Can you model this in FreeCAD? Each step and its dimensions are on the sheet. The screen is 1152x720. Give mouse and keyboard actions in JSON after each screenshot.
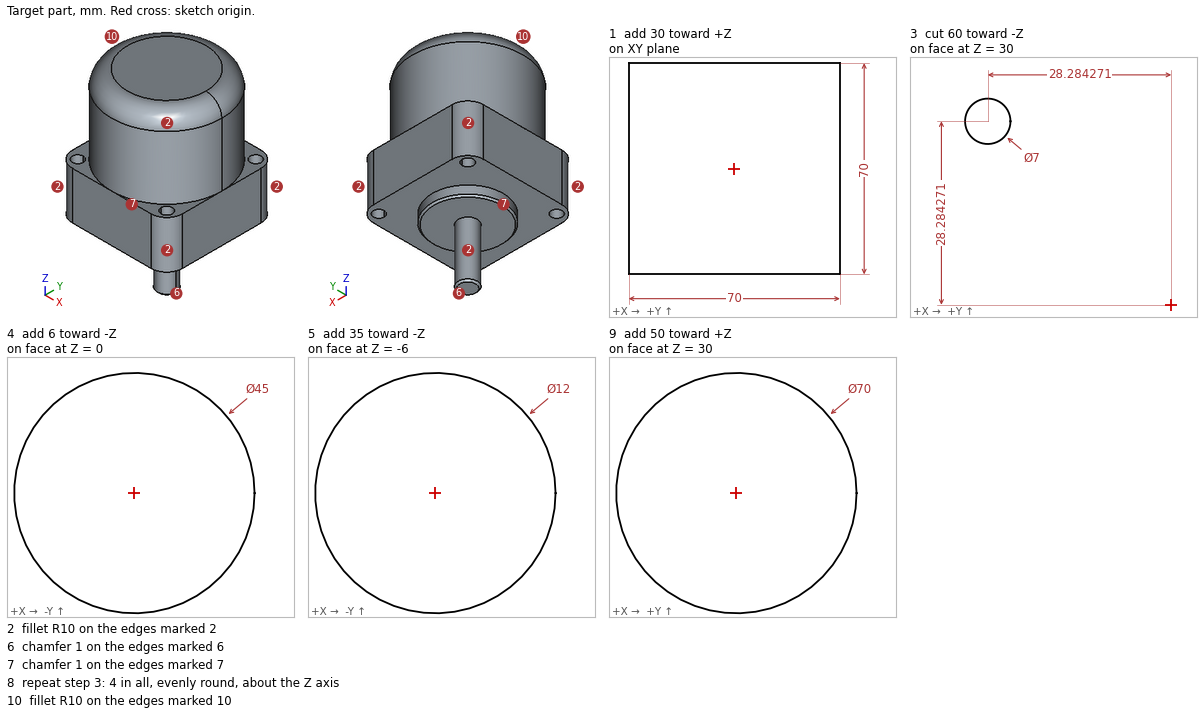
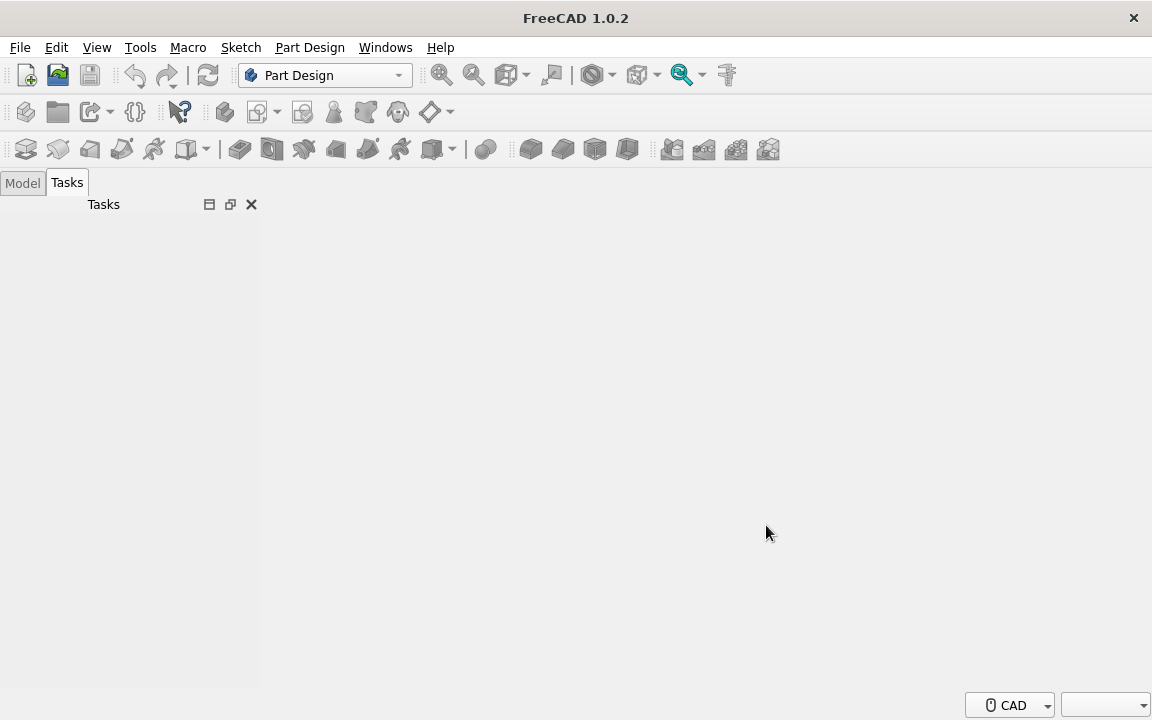
{"action": "key", "text": "ctrl+n"}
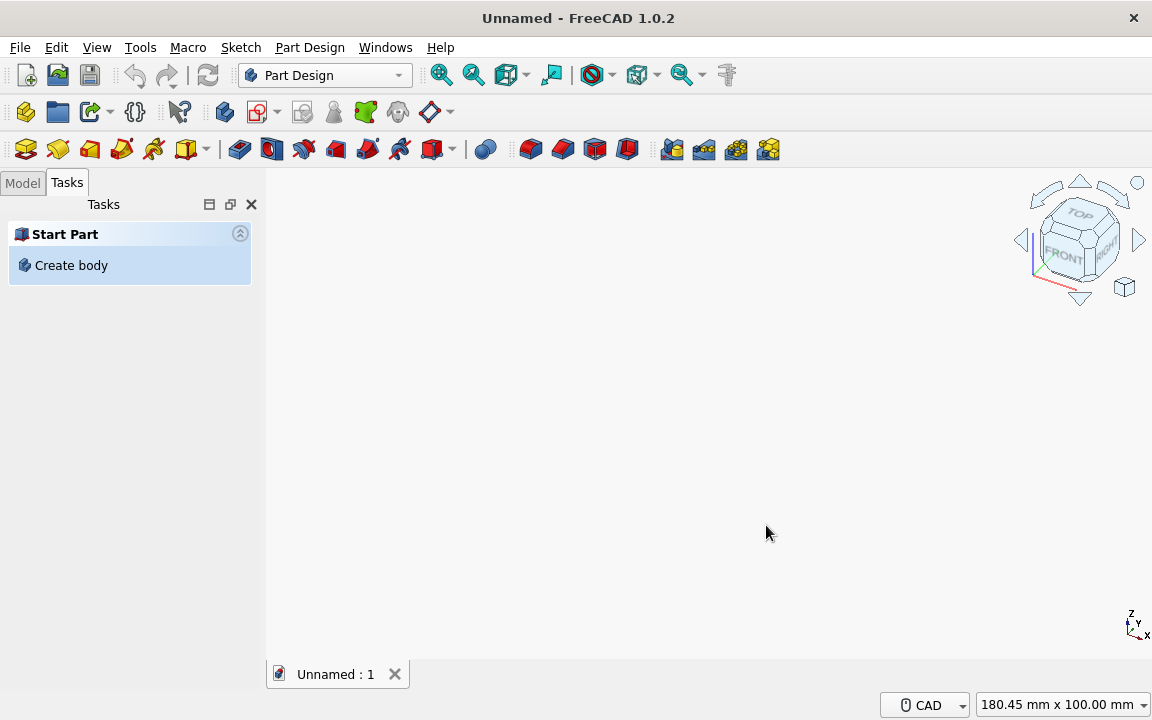
{"action": "left_click", "coordinate": [258, 112]}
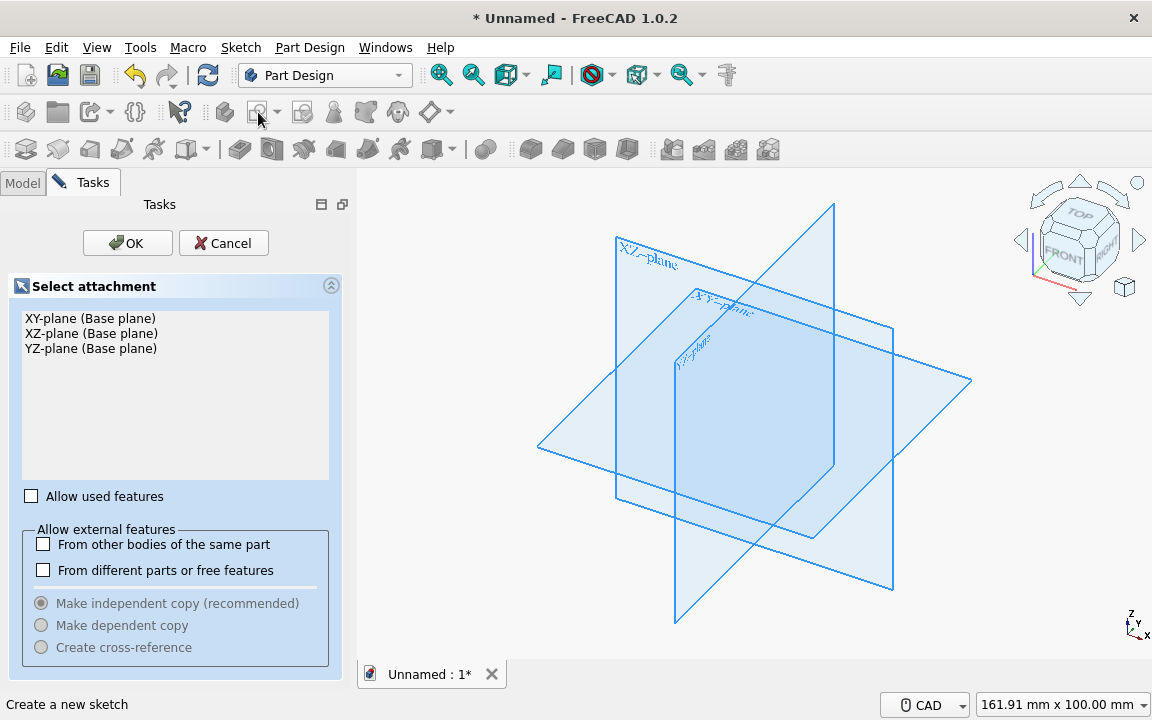
{"action": "left_click", "coordinate": [82, 318]}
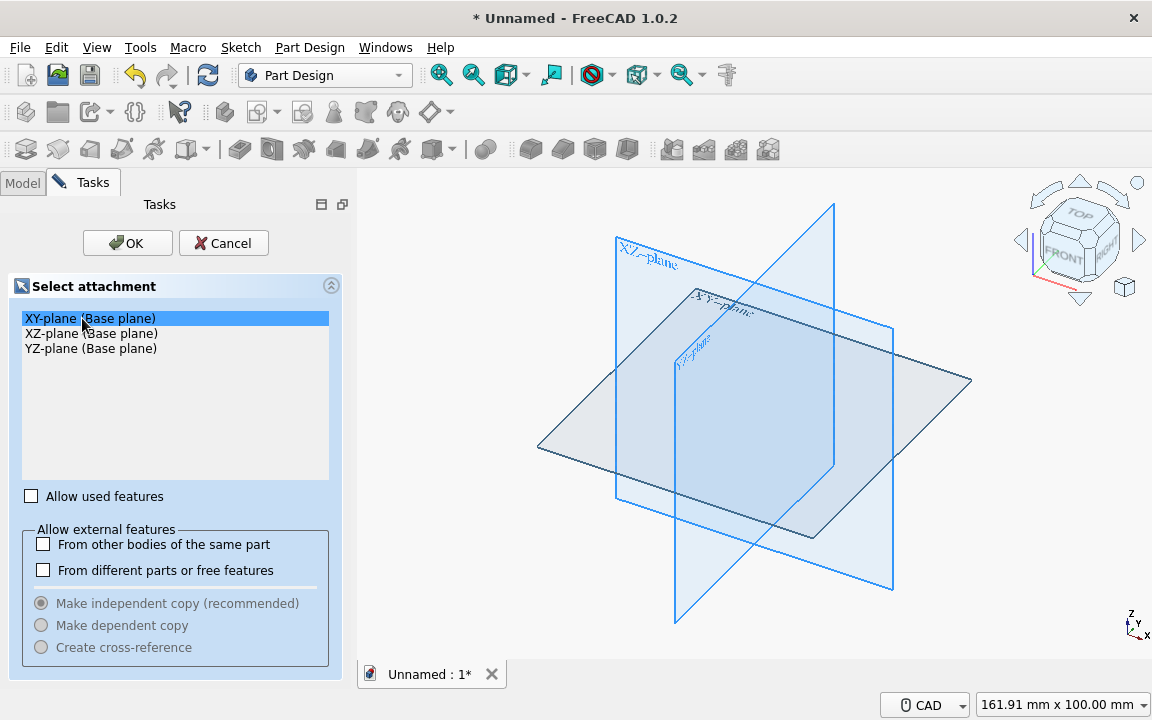
{"action": "left_click", "coordinate": [128, 243]}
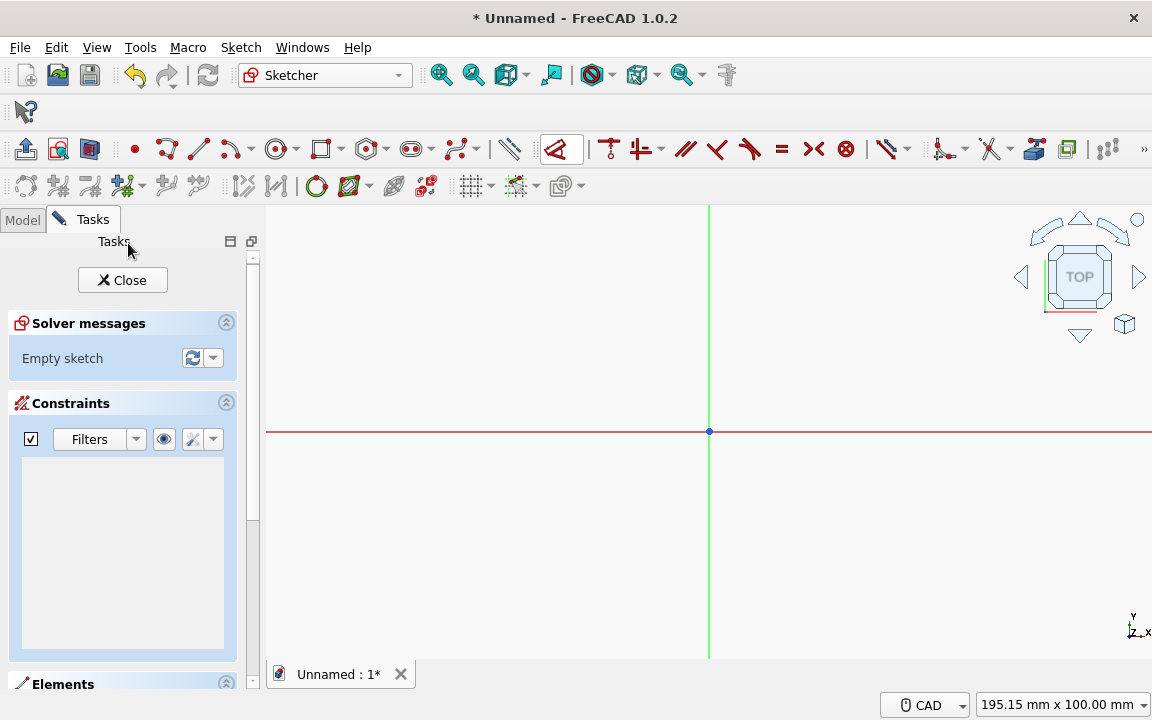
{"action": "key", "text": "g v"}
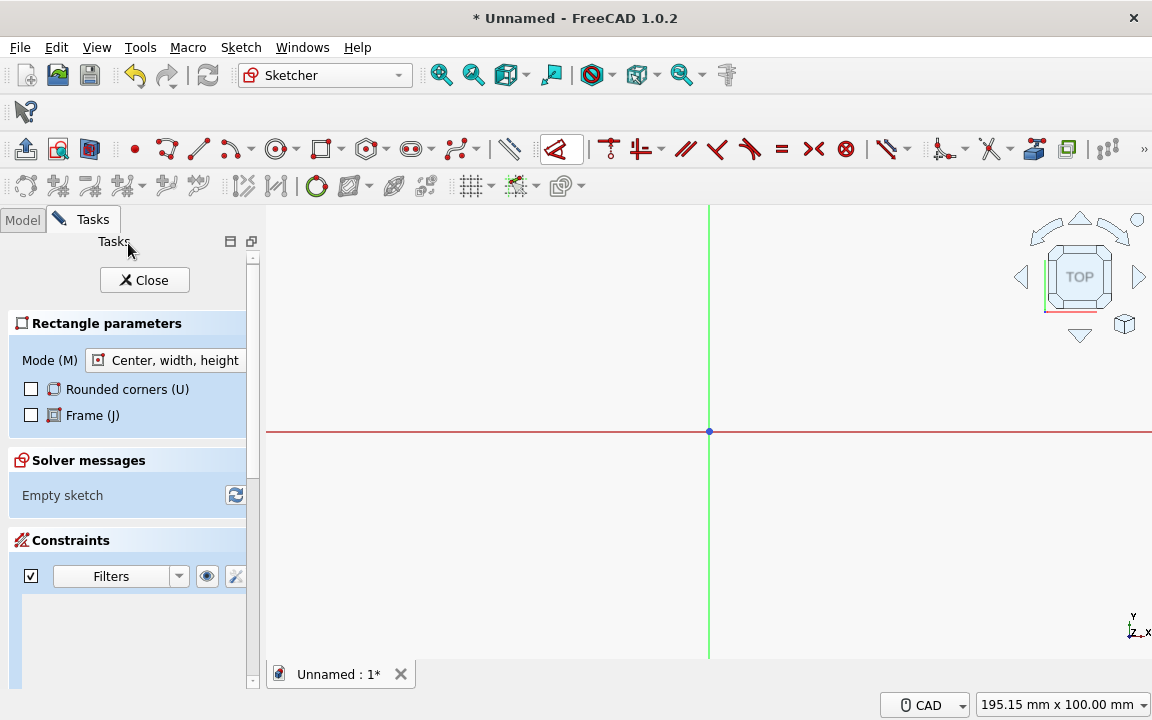
{"action": "left_click", "coordinate": [709, 432]}
{"action": "mouse_move", "coordinate": [868, 273]}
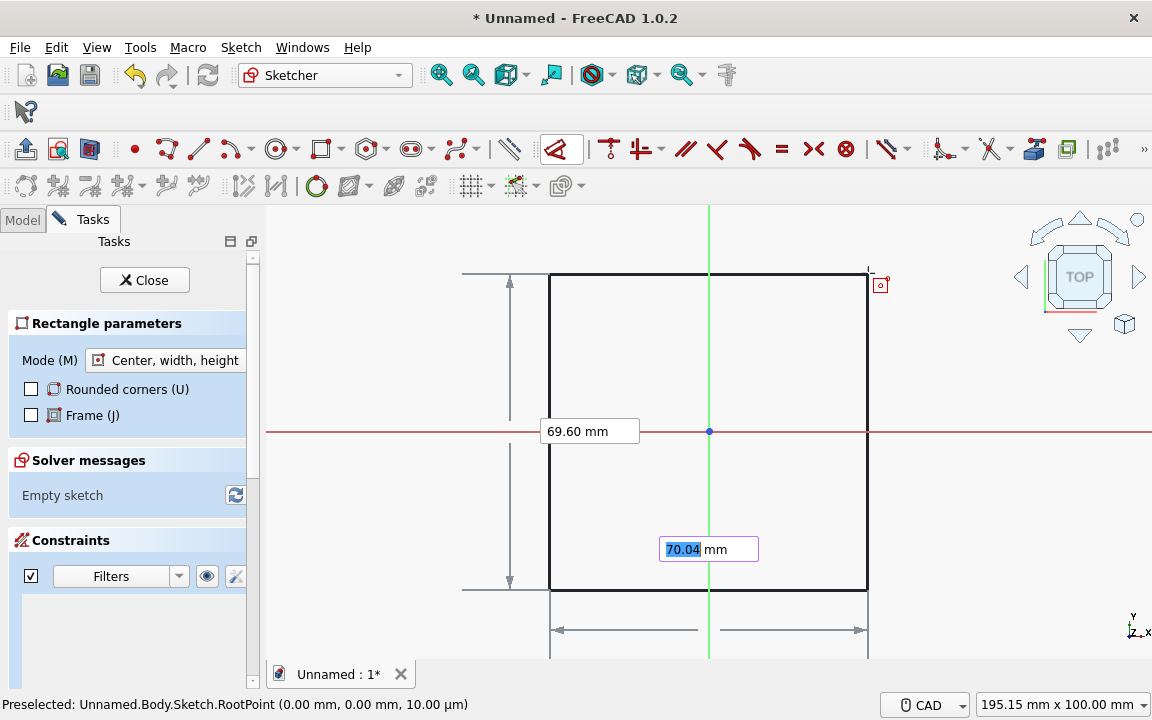
{"action": "type", "text": "70"}
{"action": "key", "text": "Tab"}
{"action": "type", "text": "70"}
{"action": "key", "text": "Return"}
{"action": "key", "text": "Escape"}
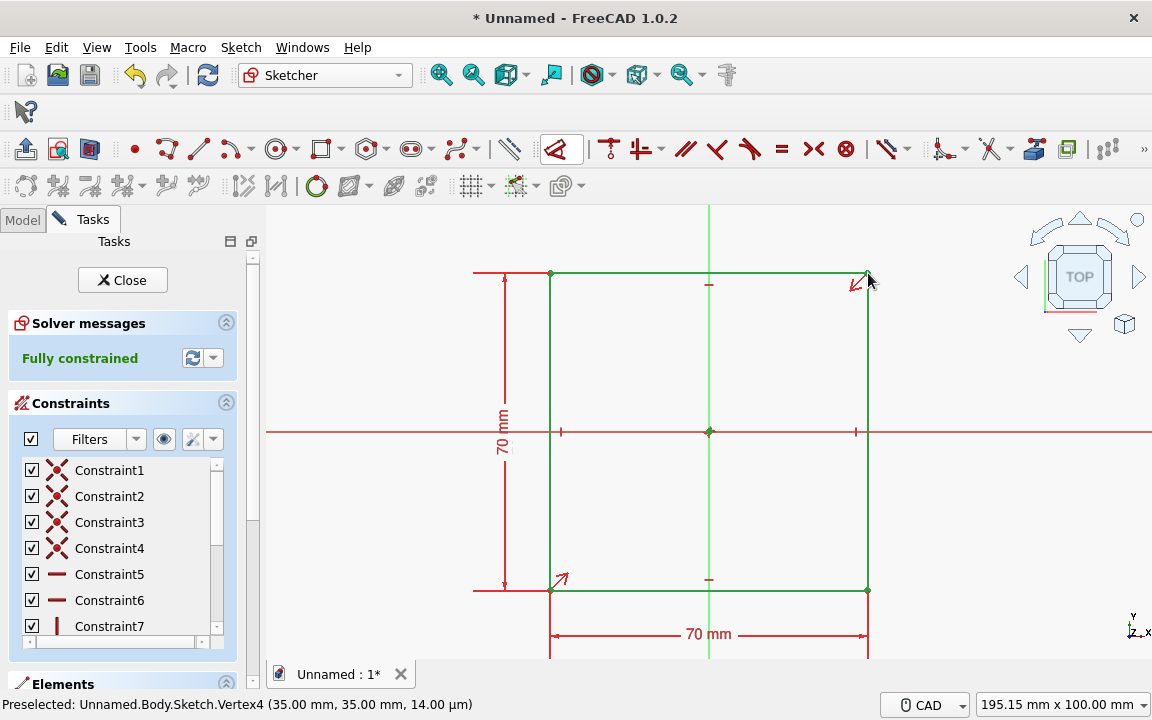
{"action": "left_click", "coordinate": [123, 280]}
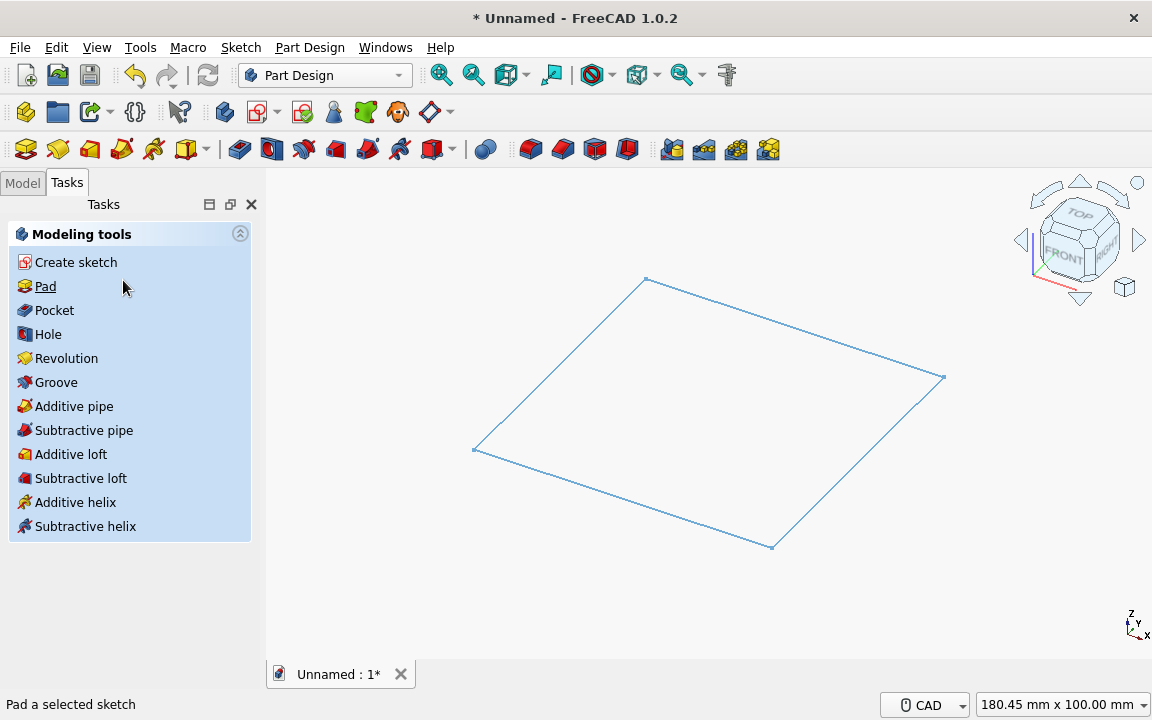
{"action": "left_click", "coordinate": [26, 150]}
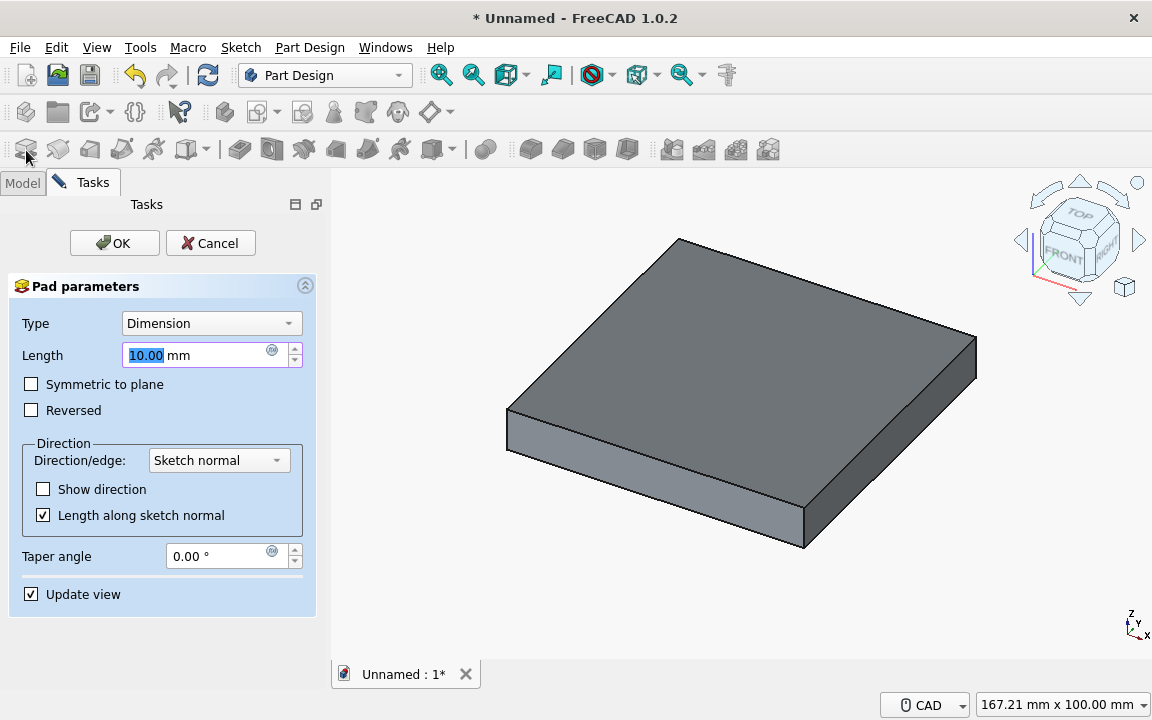
{"action": "type", "text": "30"}
{"action": "key", "text": "Tab"}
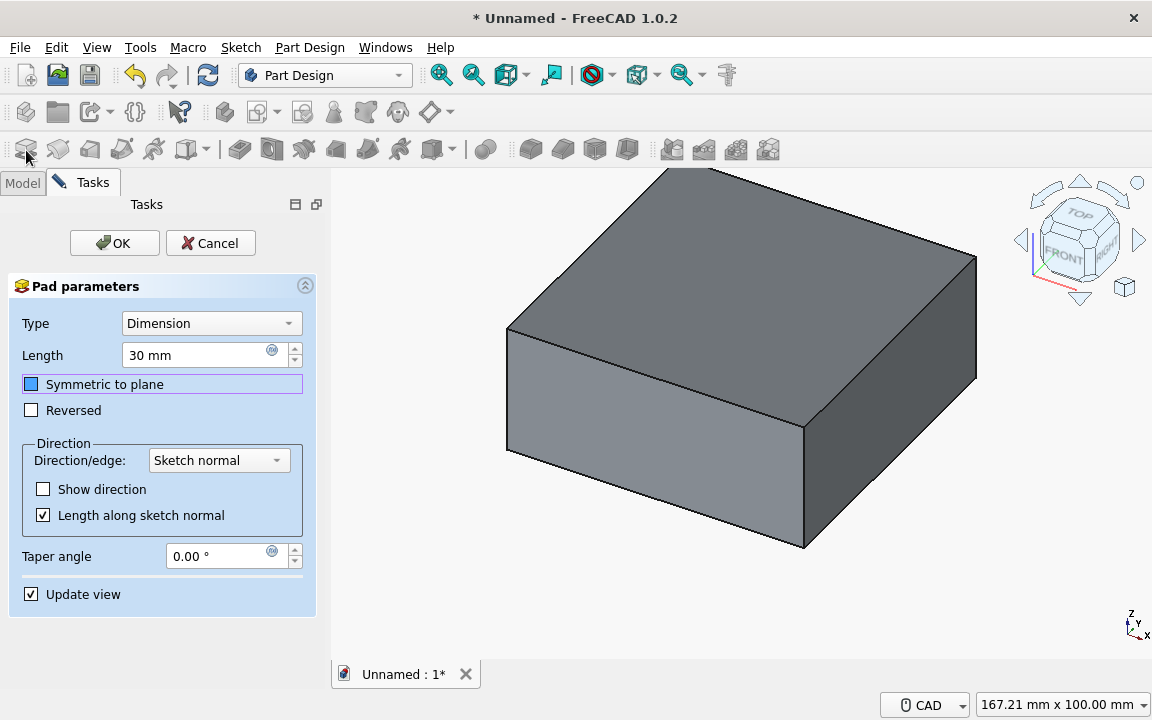
{"action": "left_click", "coordinate": [115, 243]}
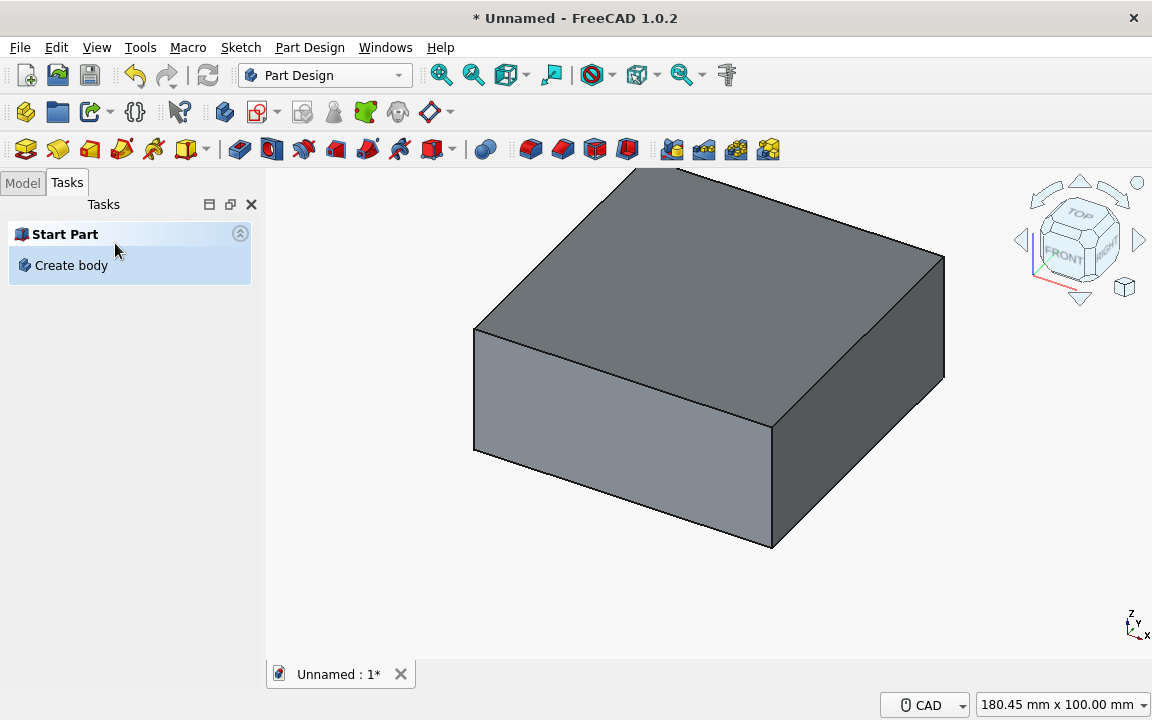
{"action": "key", "text": "v f"}